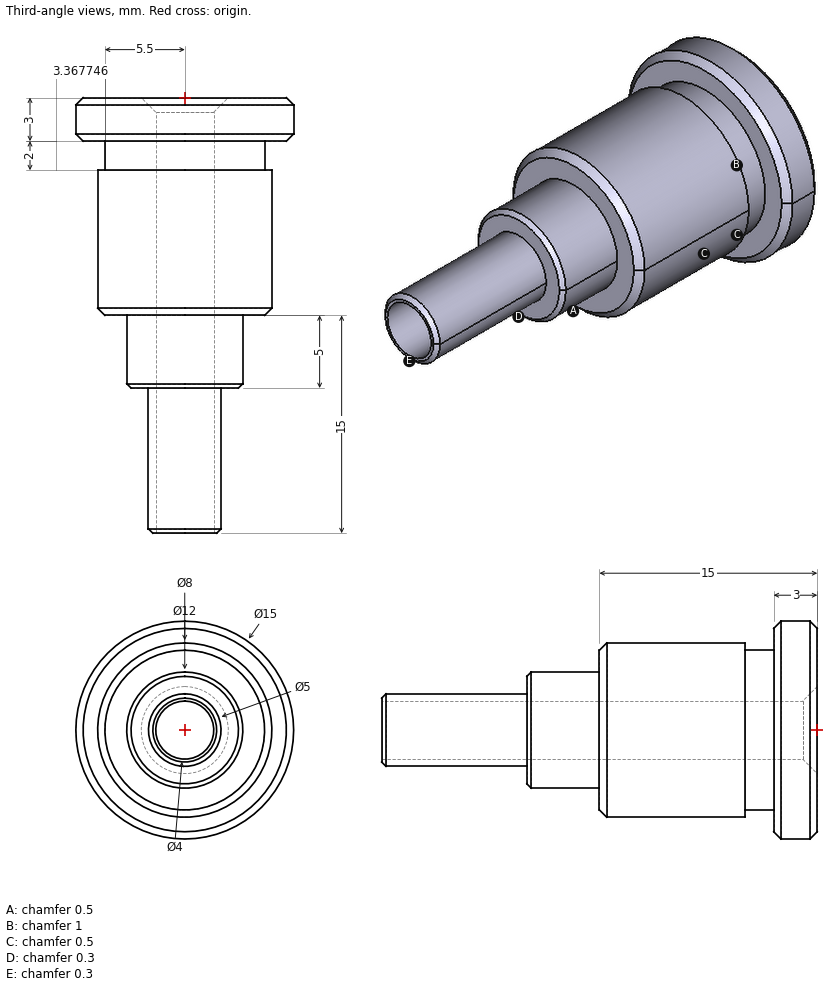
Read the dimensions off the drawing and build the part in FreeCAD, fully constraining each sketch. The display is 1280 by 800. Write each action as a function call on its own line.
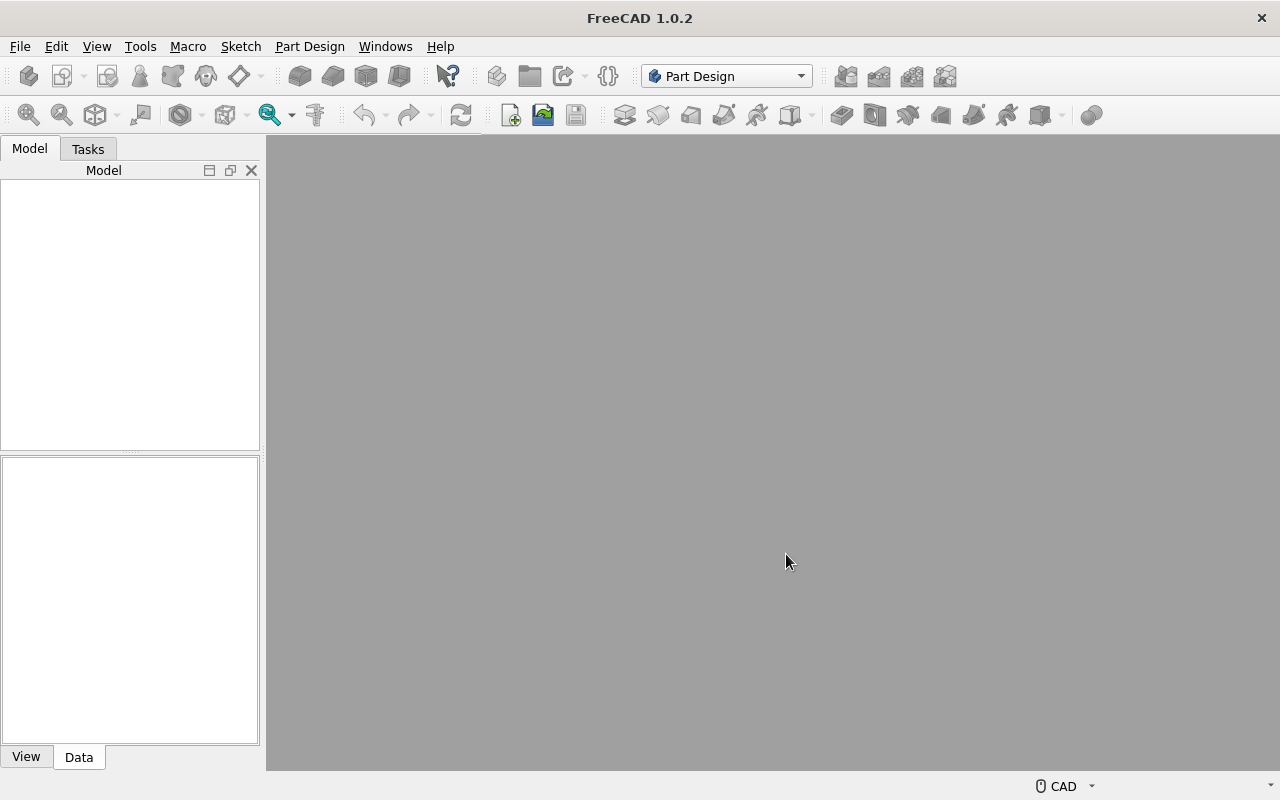
click(510, 116)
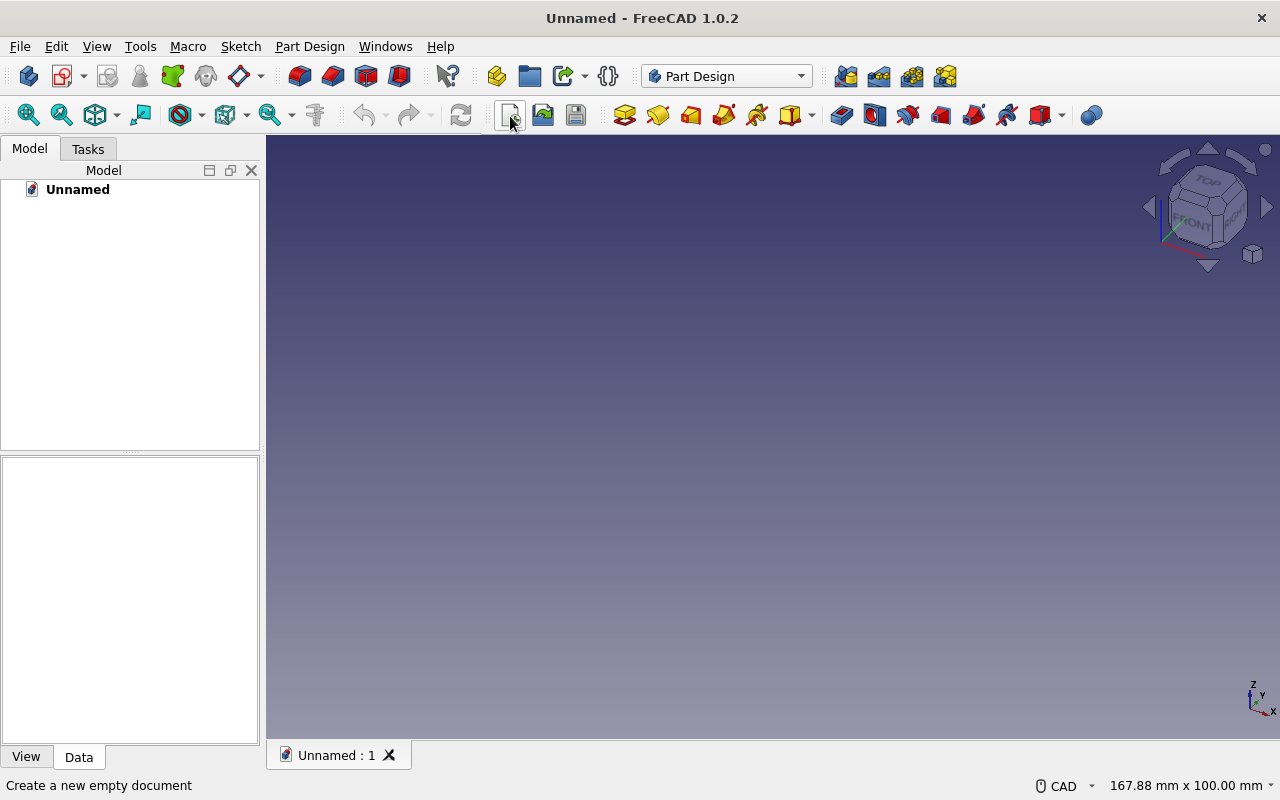
click(62, 76)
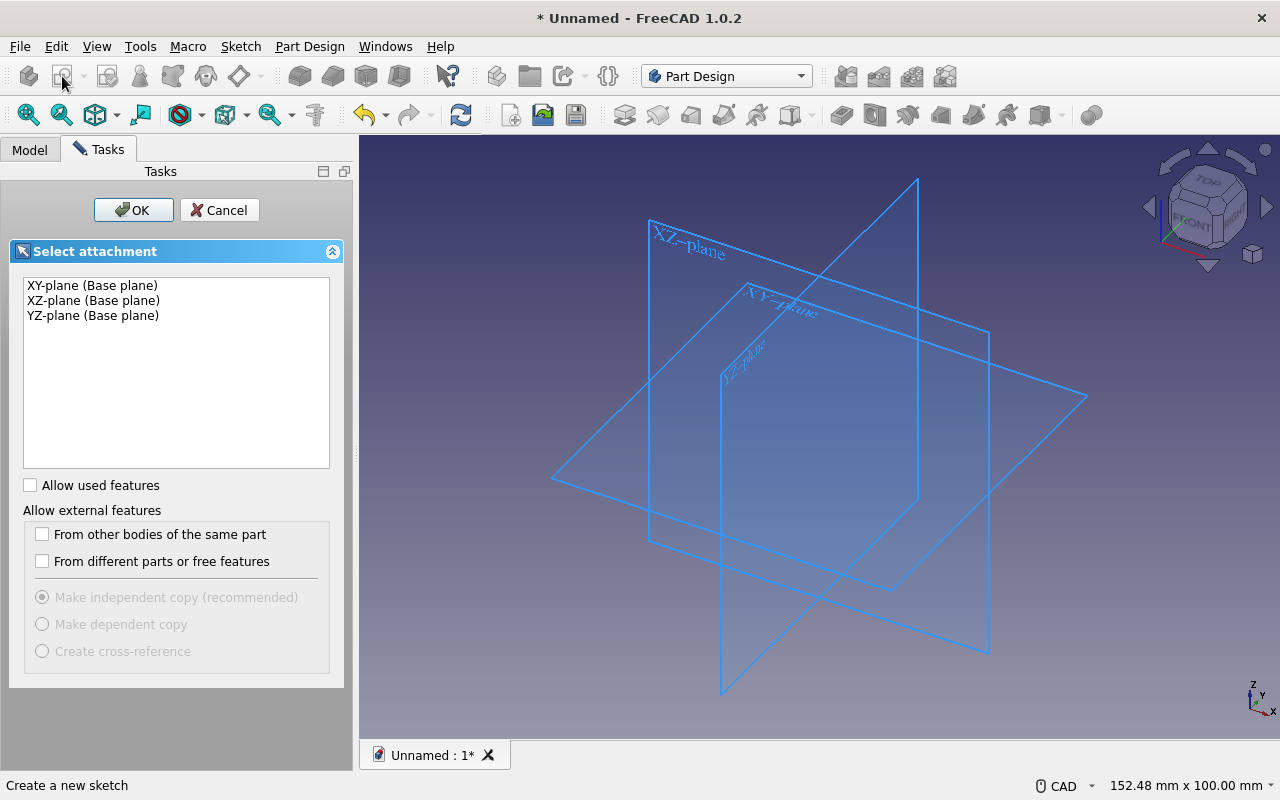
click(84, 300)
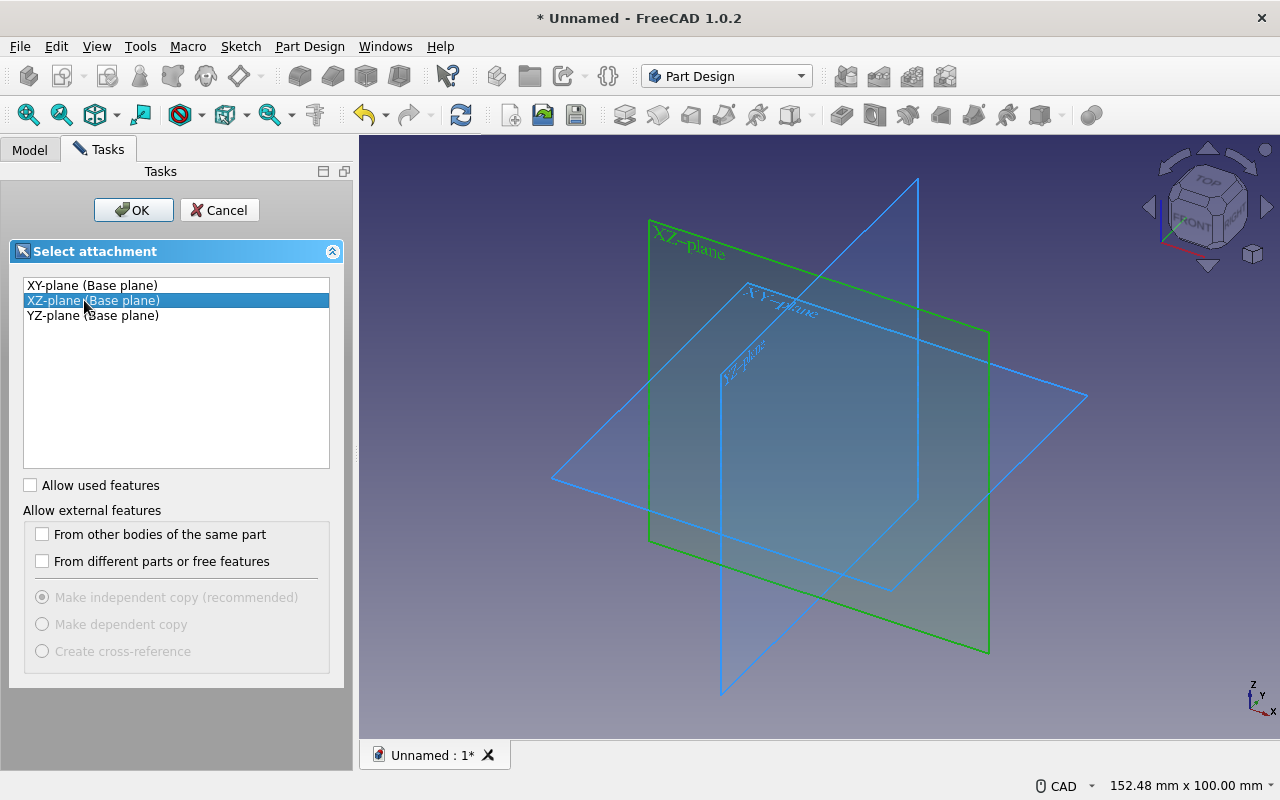
click(134, 210)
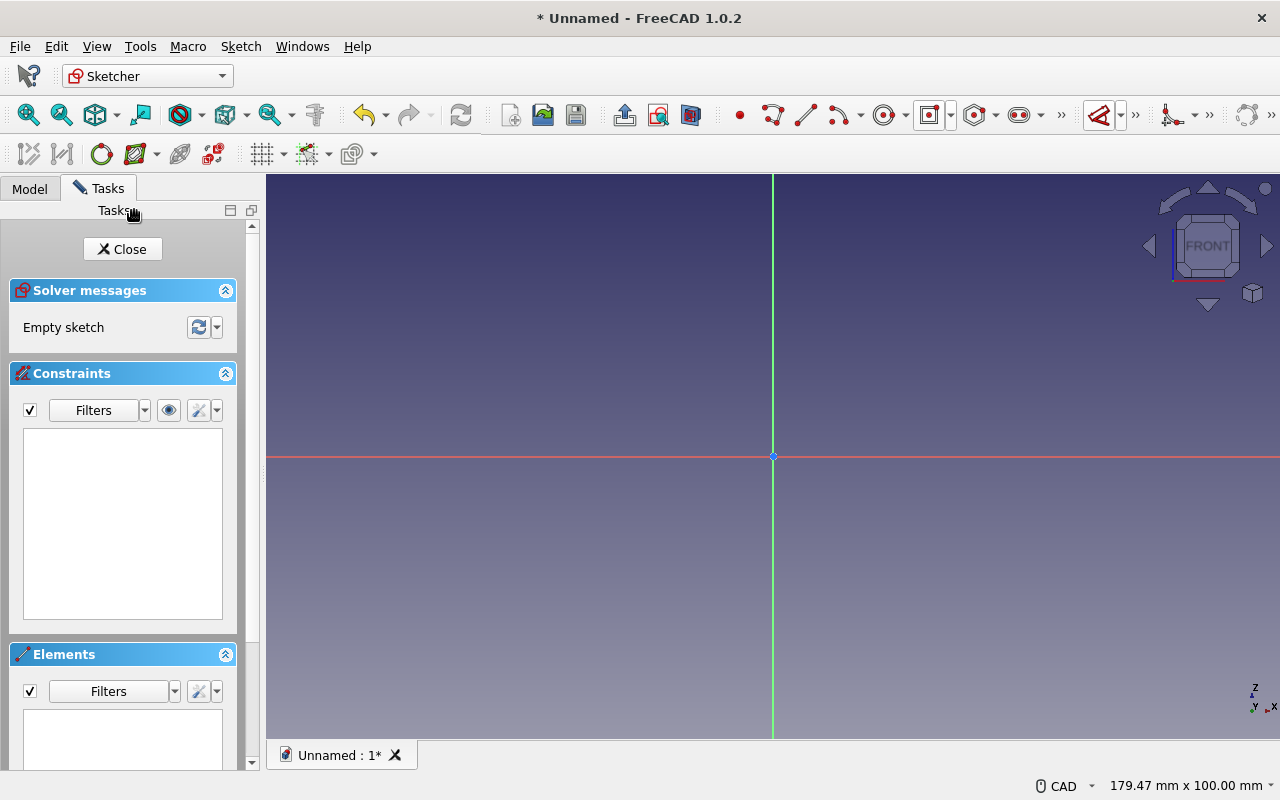
scroll(790, 456, up, 8)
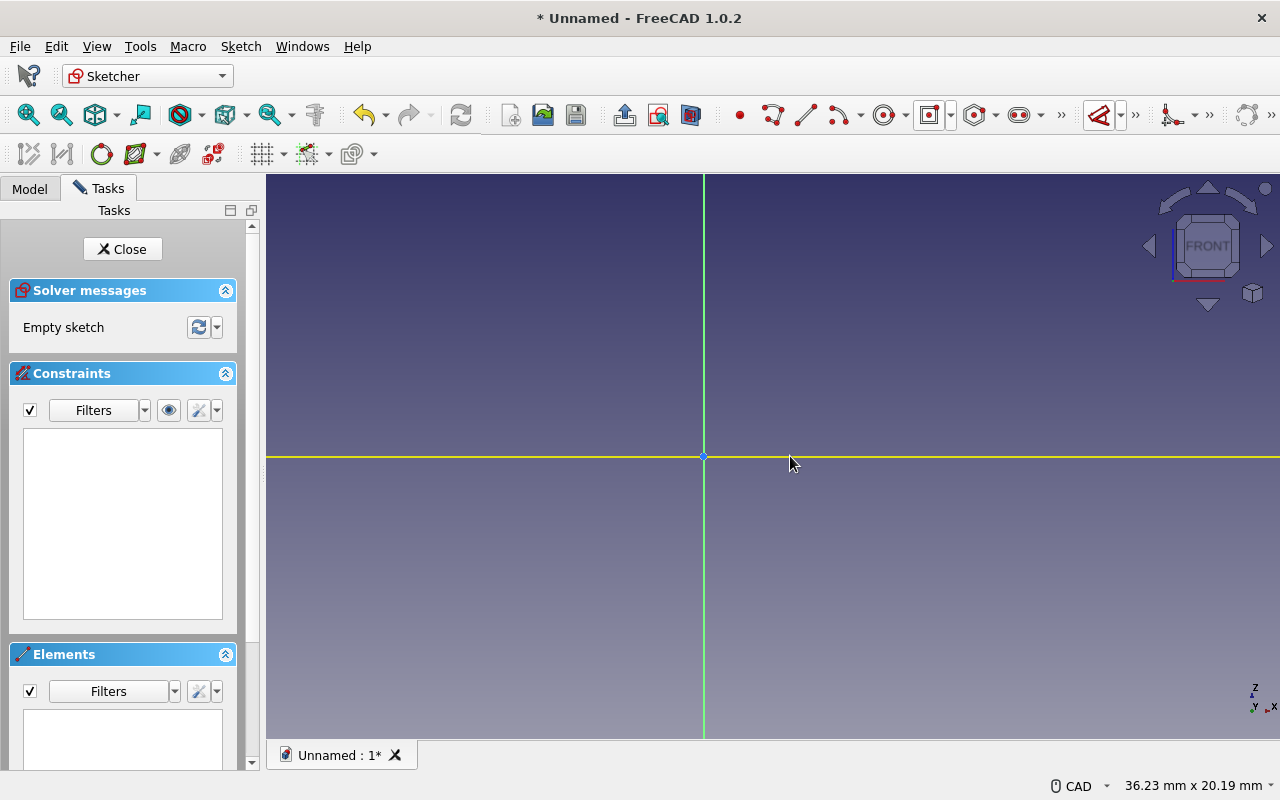
click(884, 116)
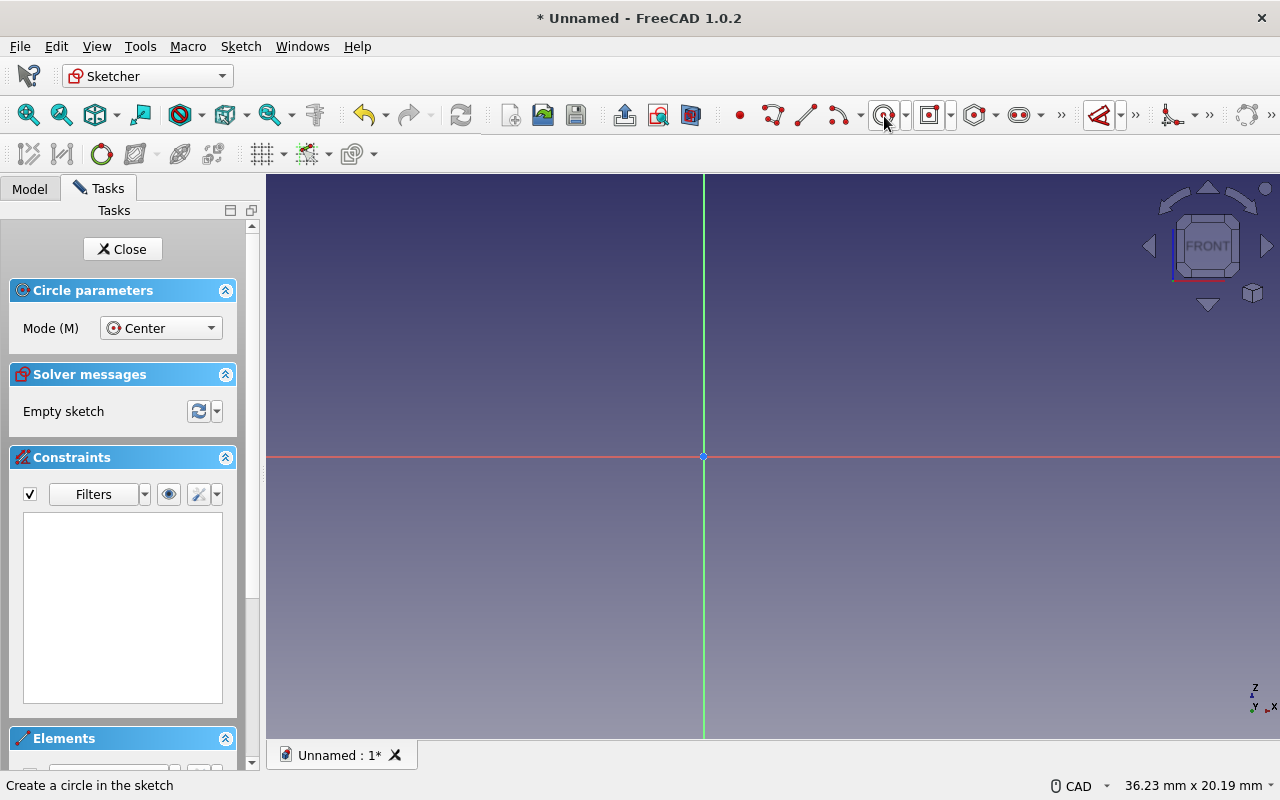
click(704, 456)
move(822, 338)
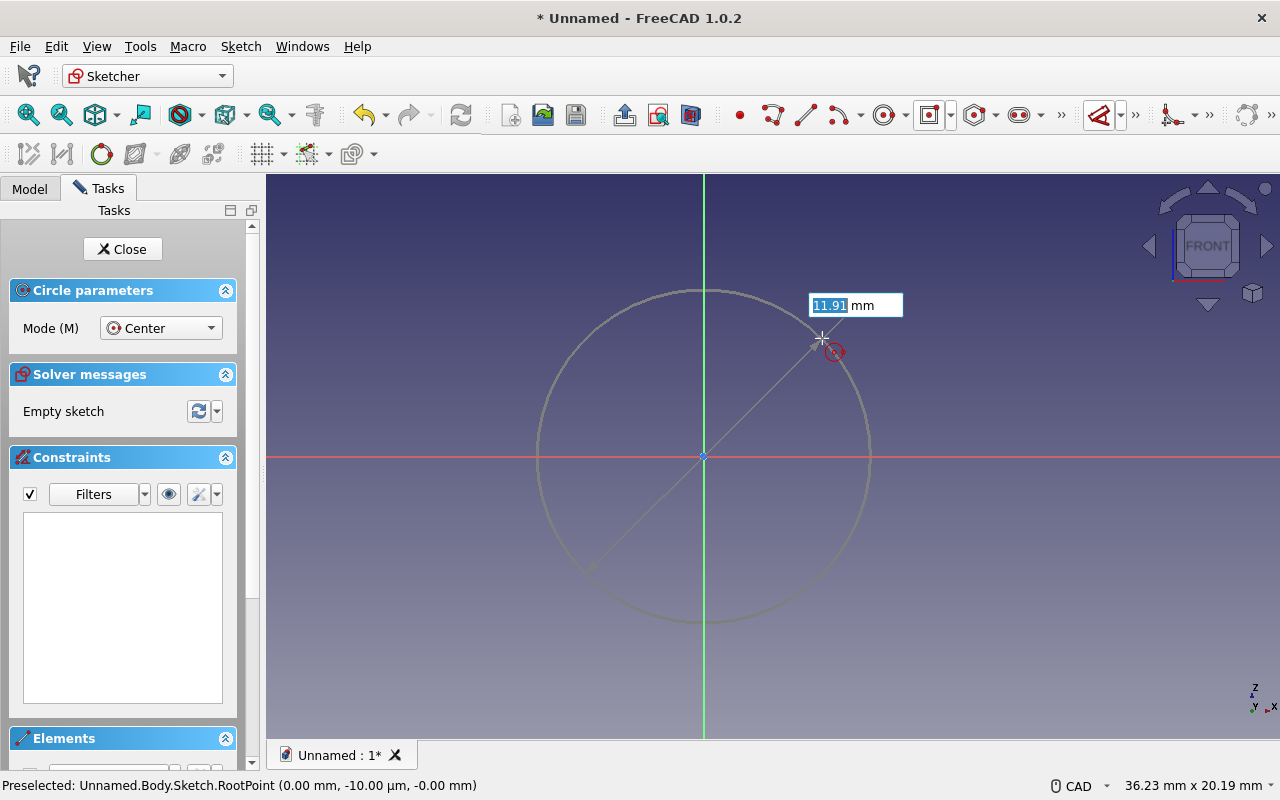
text(12)
key(Return)
key(Escape)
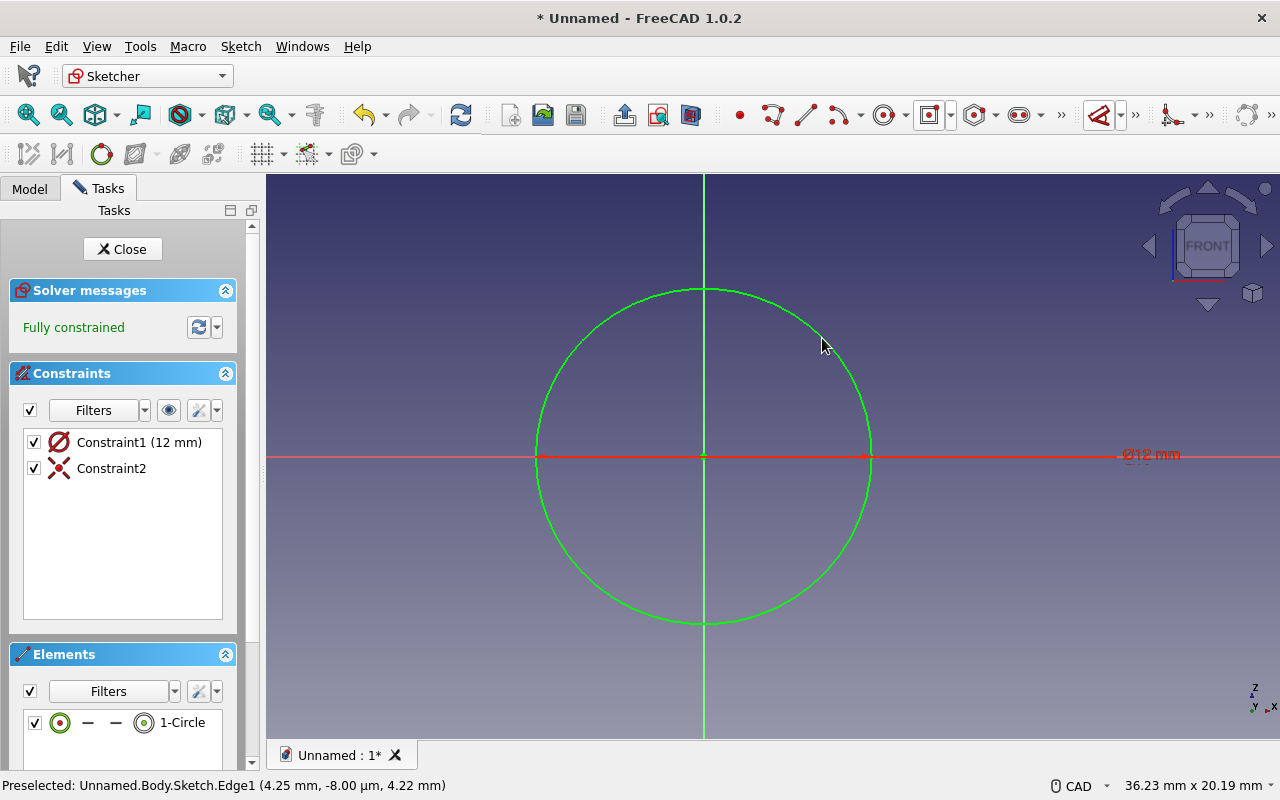
click(123, 249)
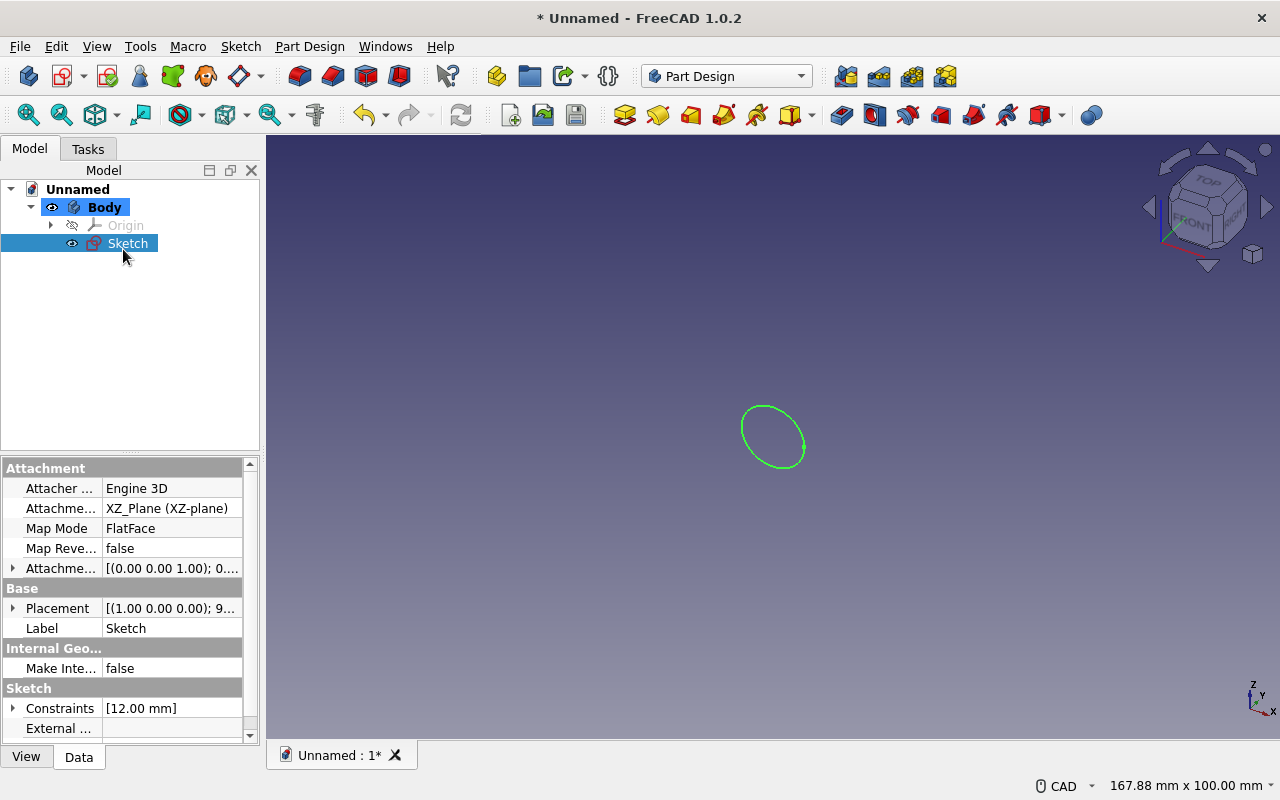
click(625, 116)